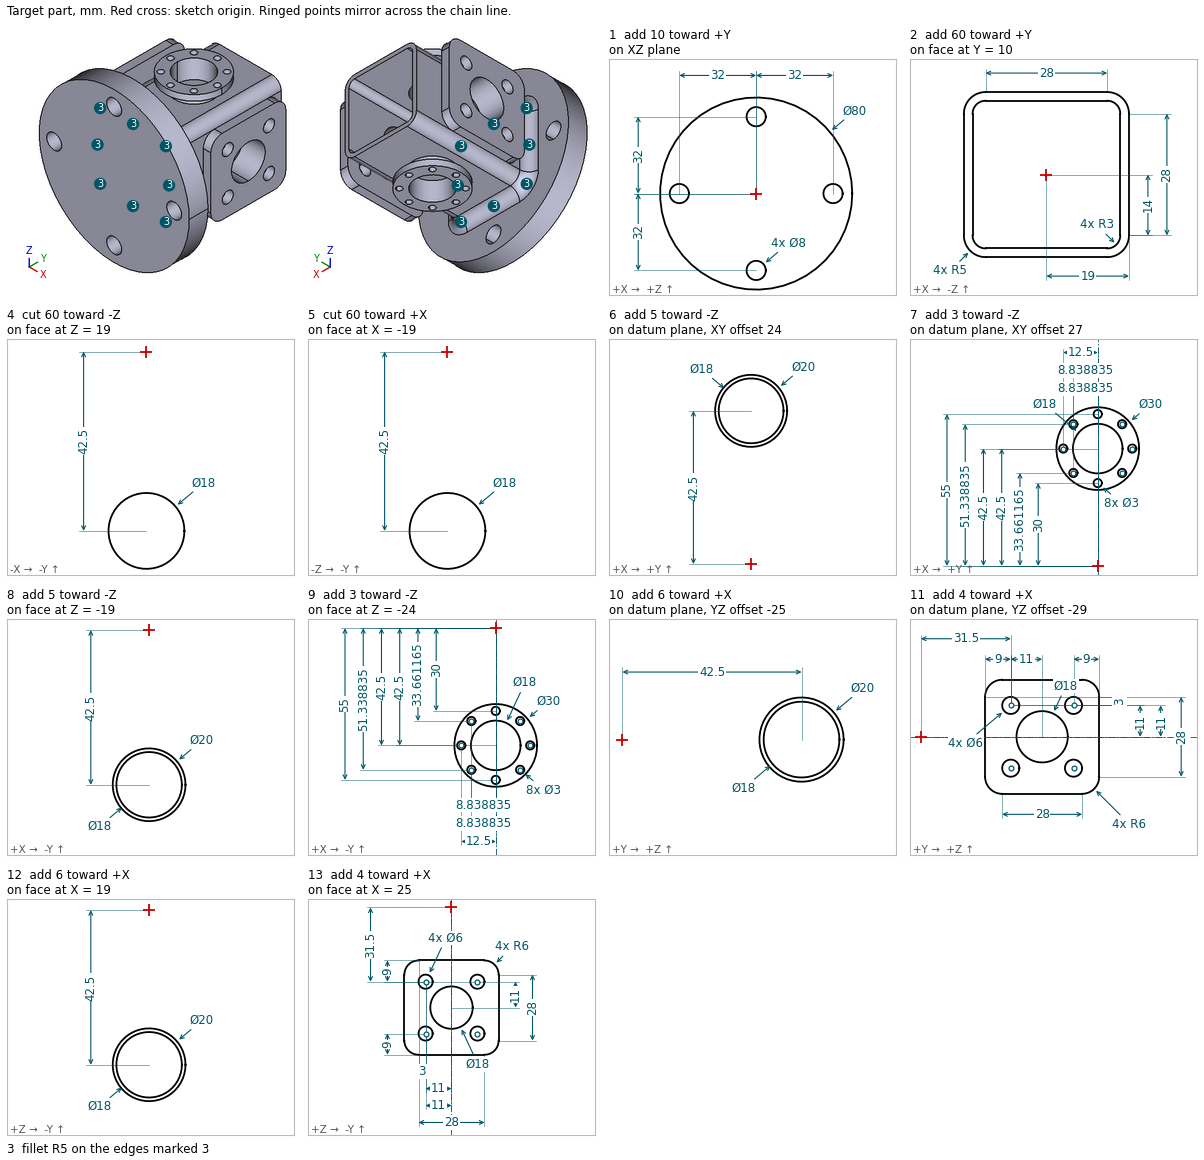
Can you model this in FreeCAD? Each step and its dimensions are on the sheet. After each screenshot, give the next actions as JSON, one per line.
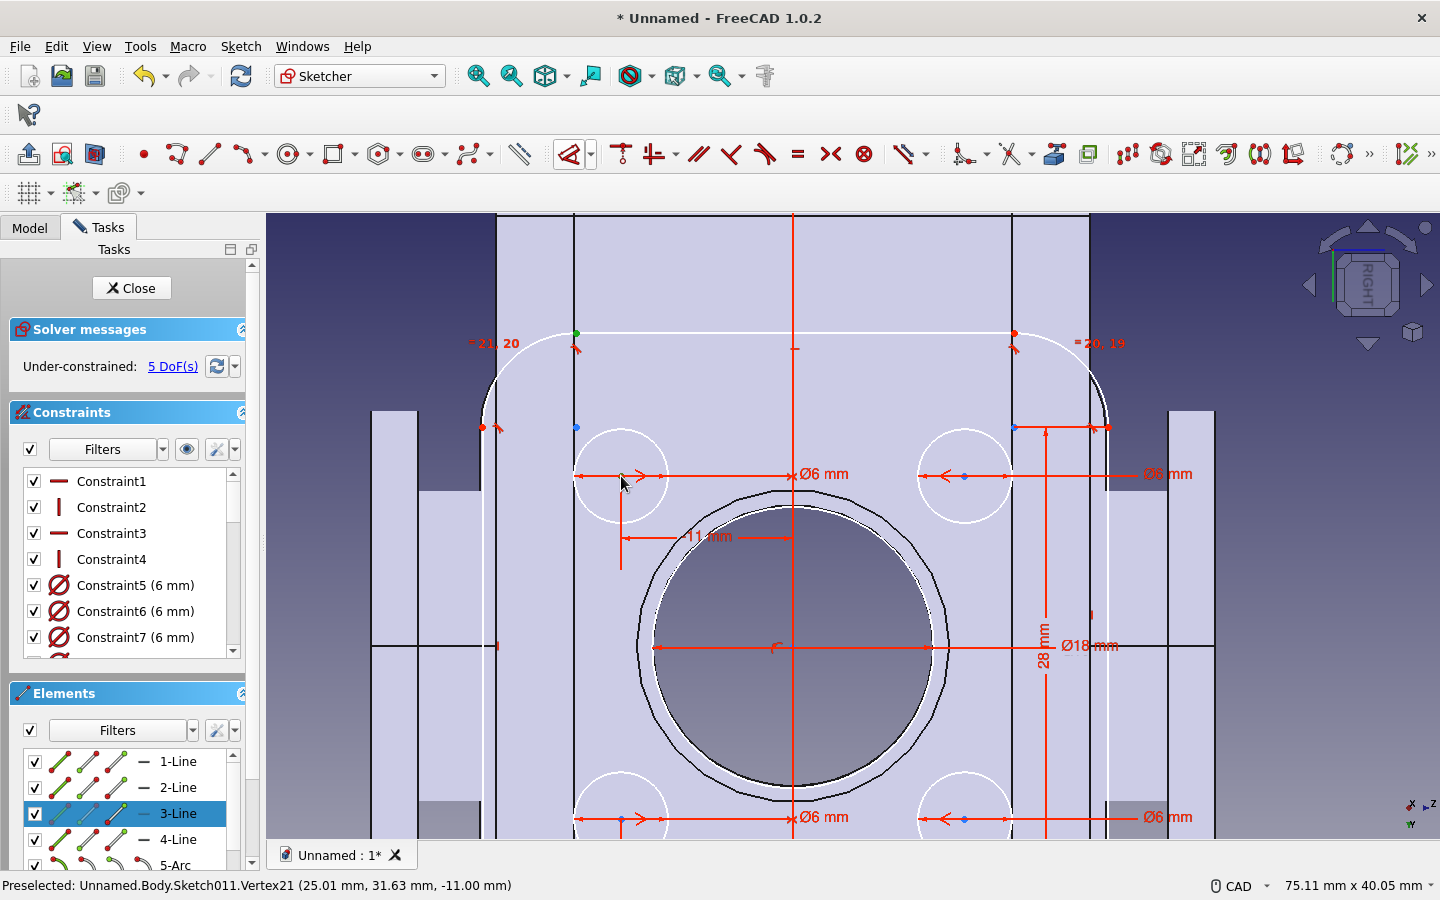
{"action": "key", "text": "l"}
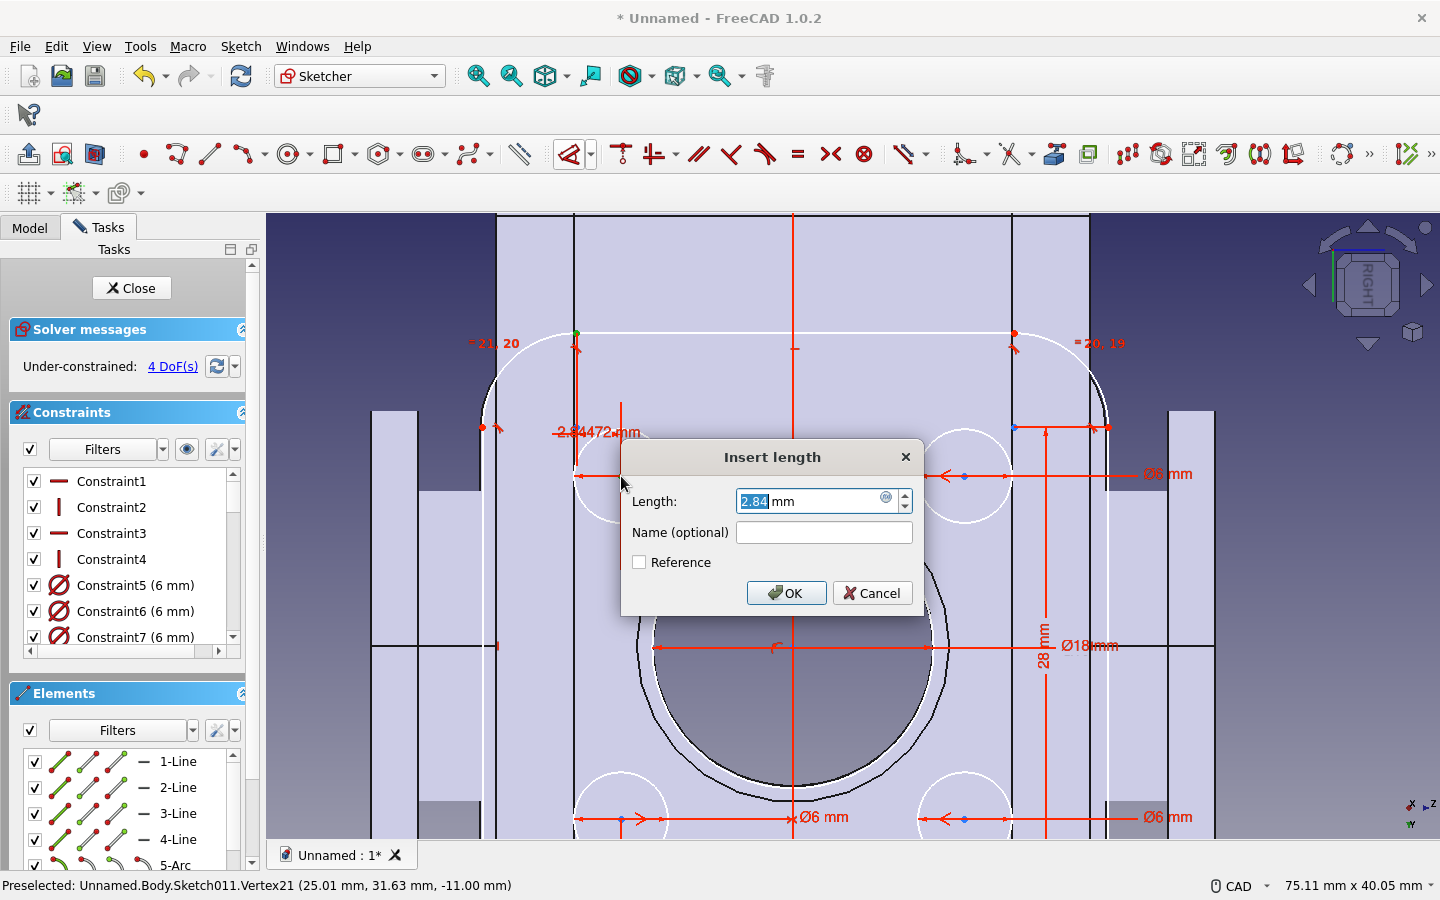
{"action": "type", "text": "3"}
{"action": "key", "text": "Return"}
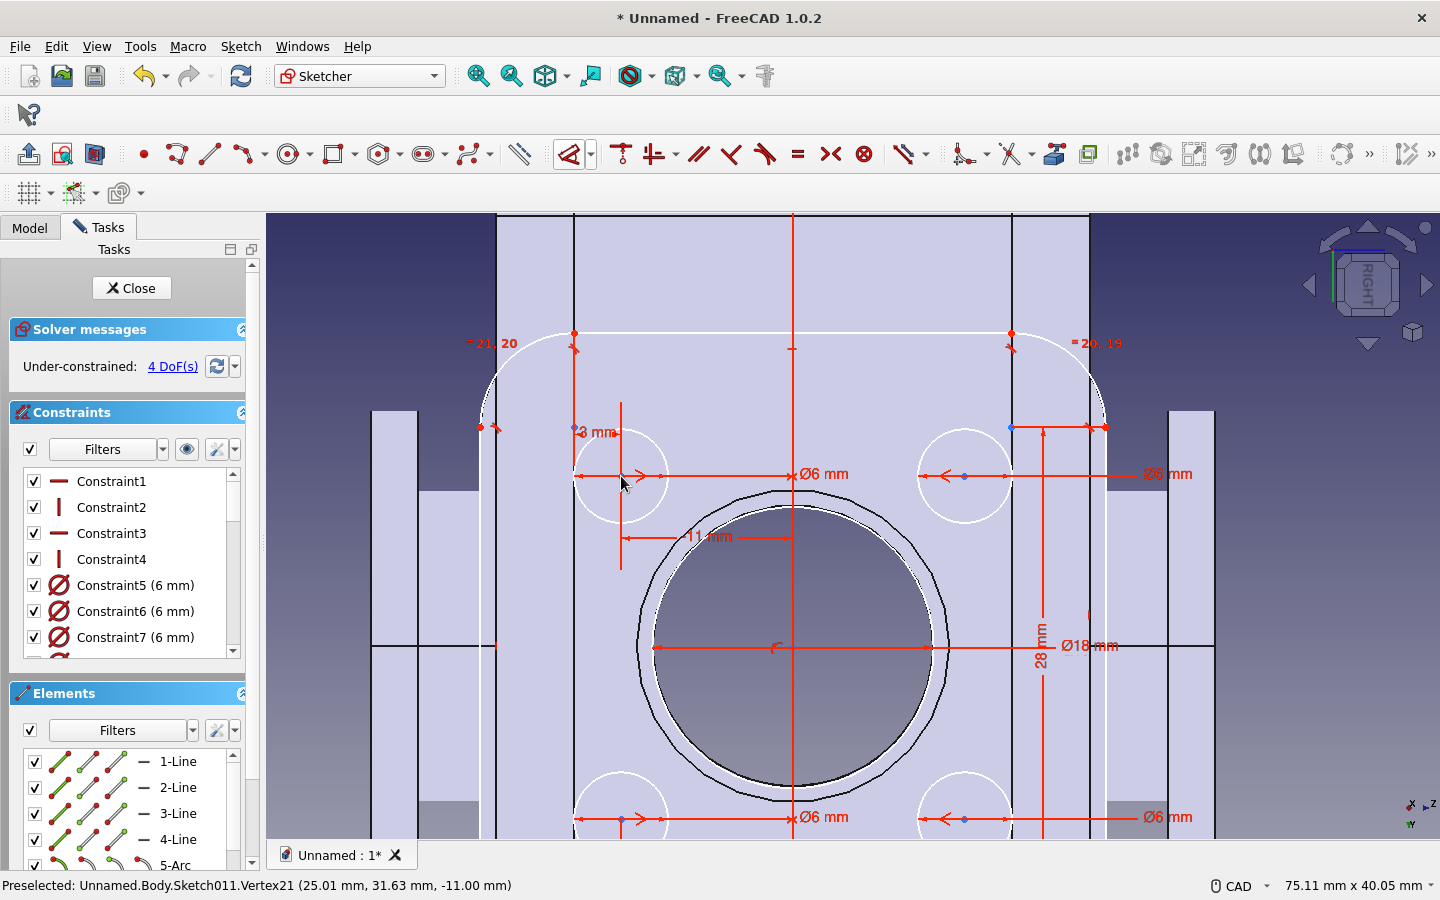
{"action": "left_click", "coordinate": [574, 333]}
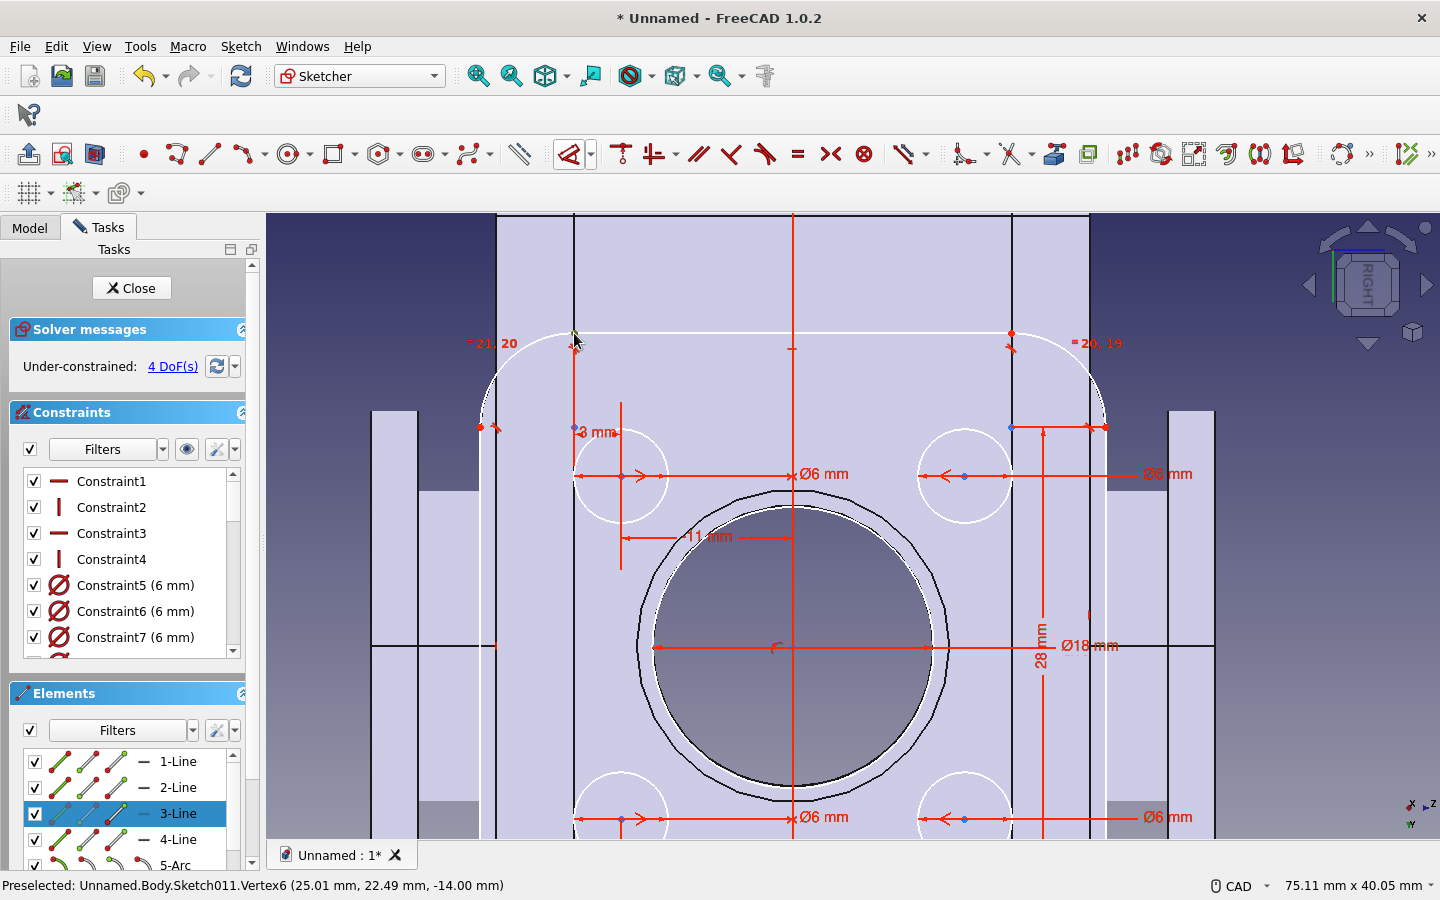
{"action": "left_click", "coordinate": [621, 476]}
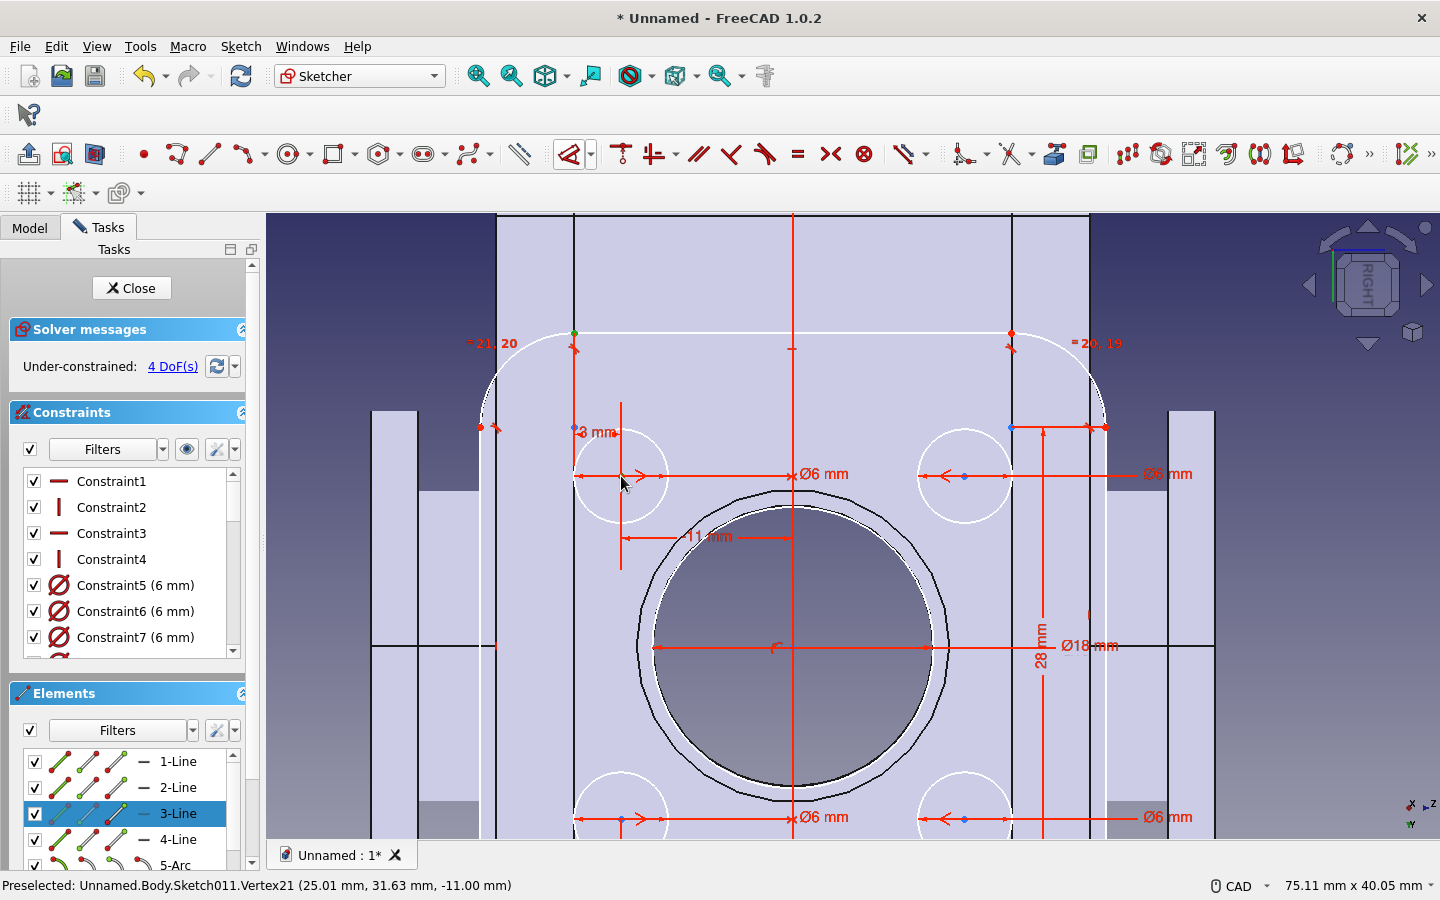
{"action": "key", "text": "i"}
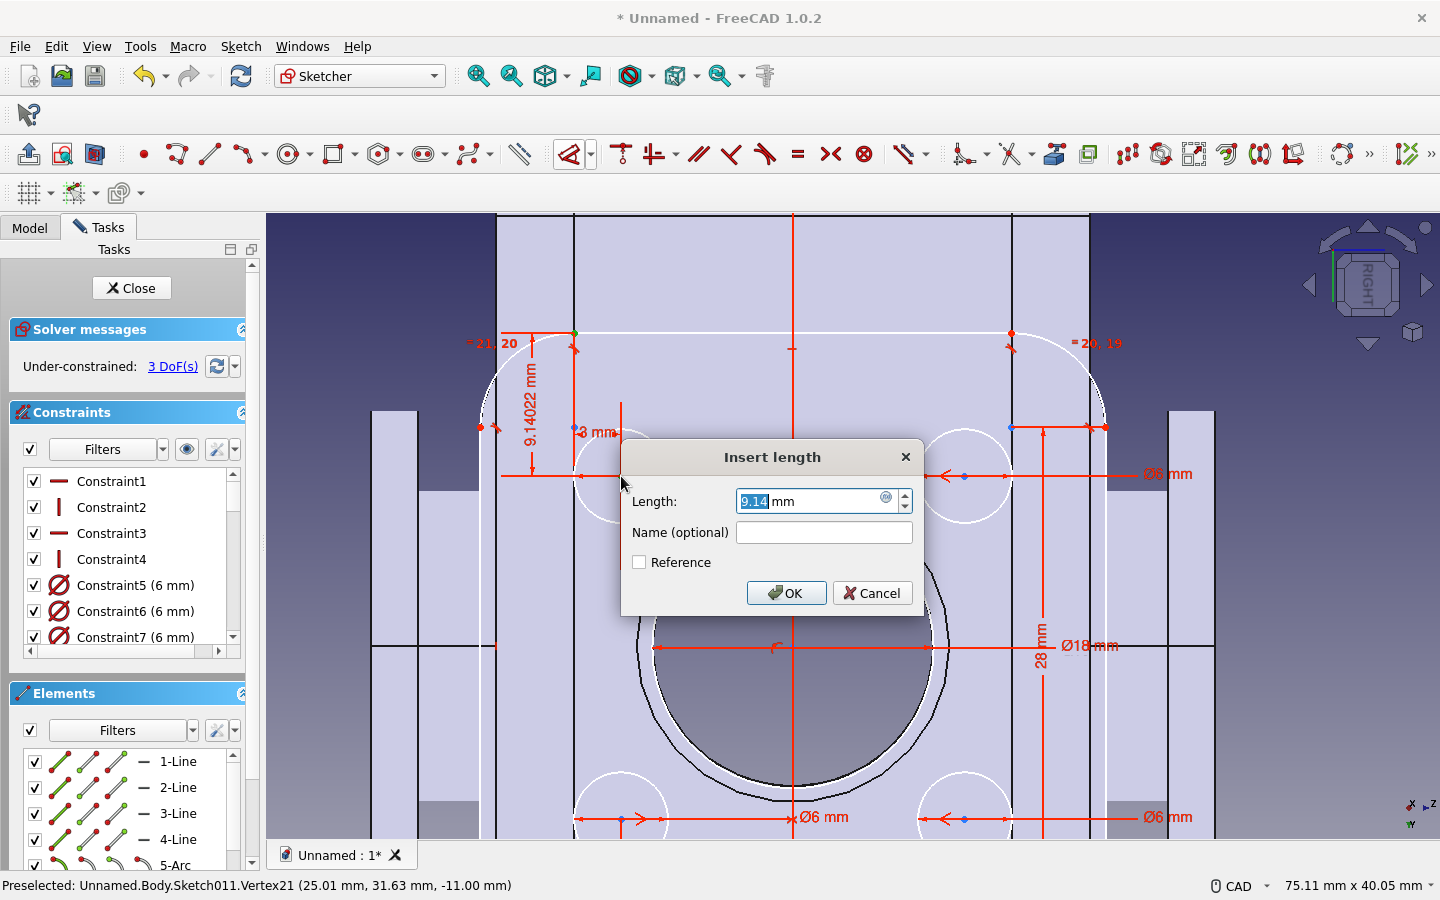
{"action": "type", "text": "9"}
{"action": "key", "text": "Return"}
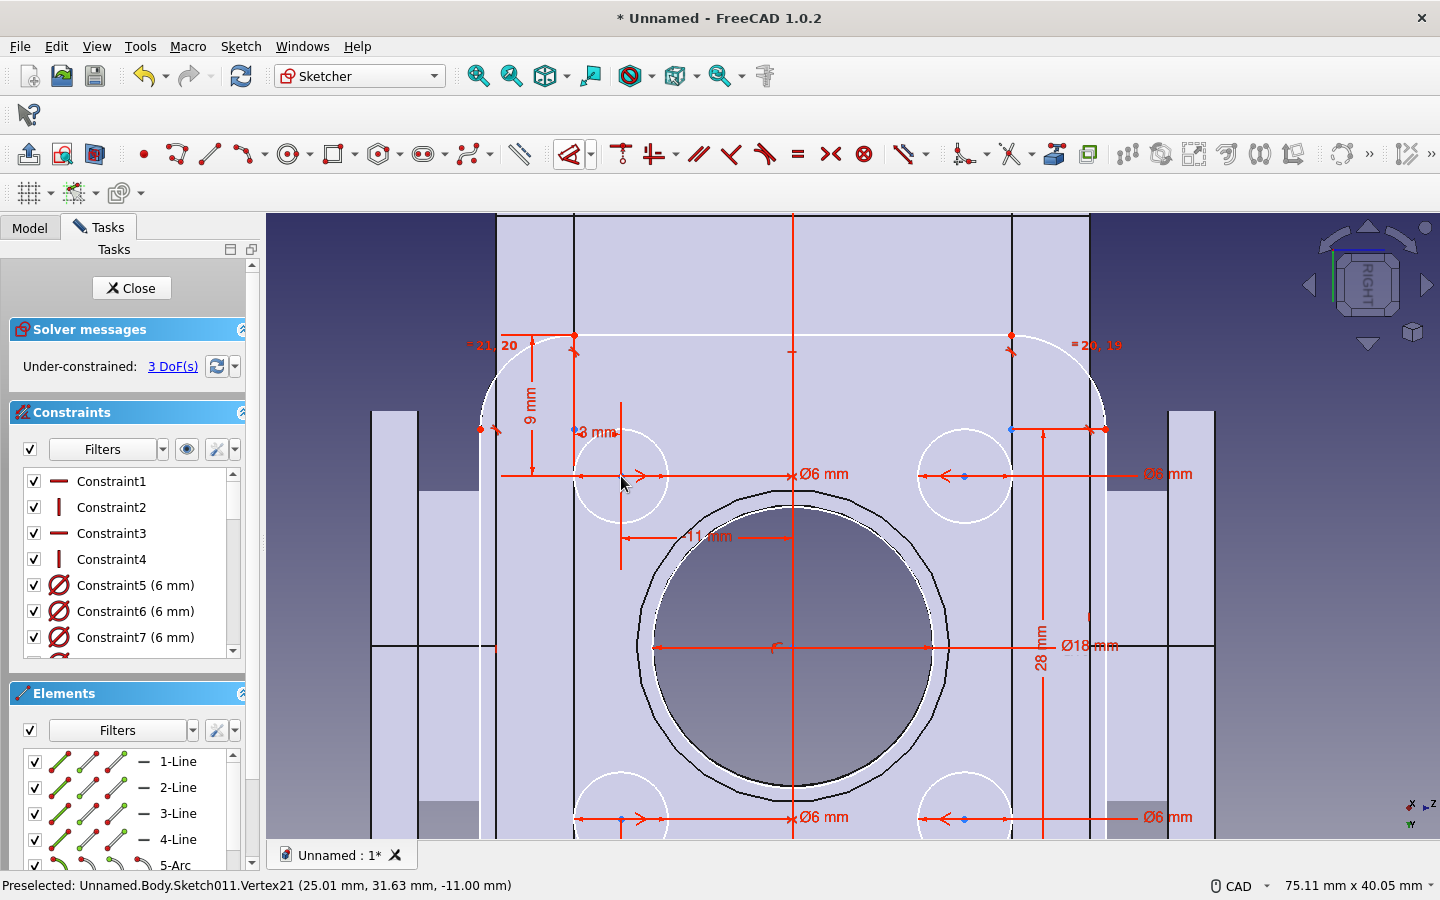
{"action": "scroll", "coordinate": [778, 572], "scroll_direction": "down", "scroll_amount": 4}